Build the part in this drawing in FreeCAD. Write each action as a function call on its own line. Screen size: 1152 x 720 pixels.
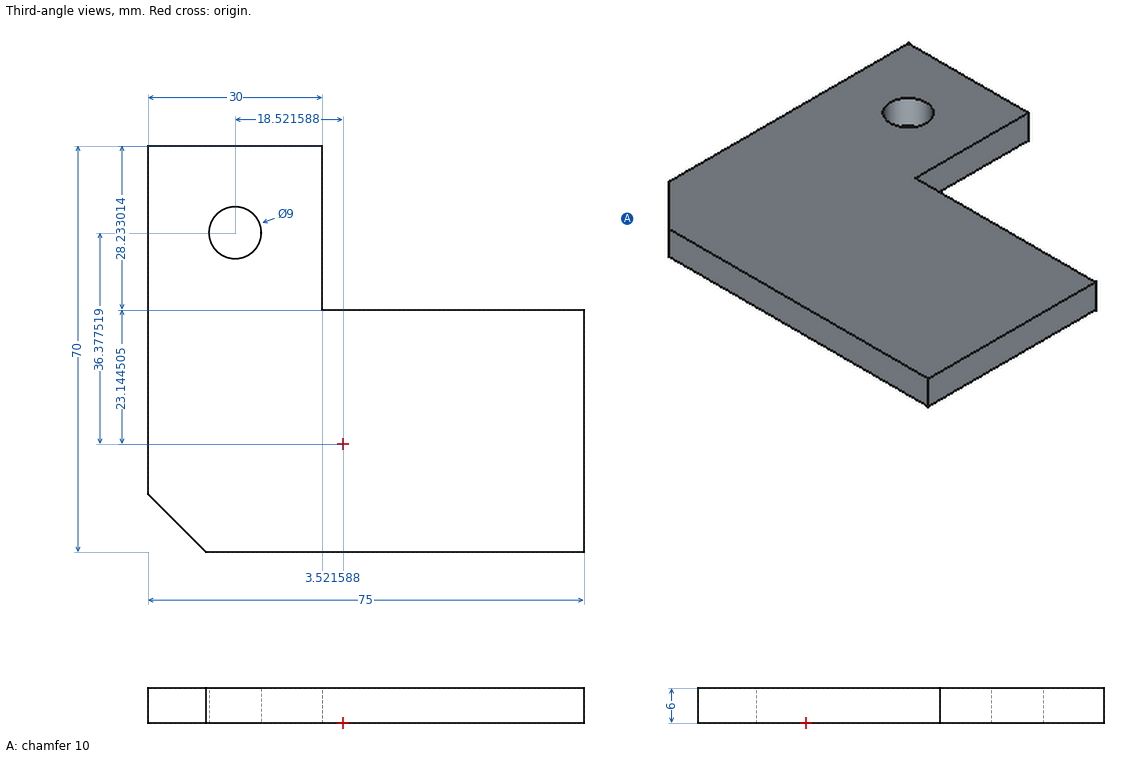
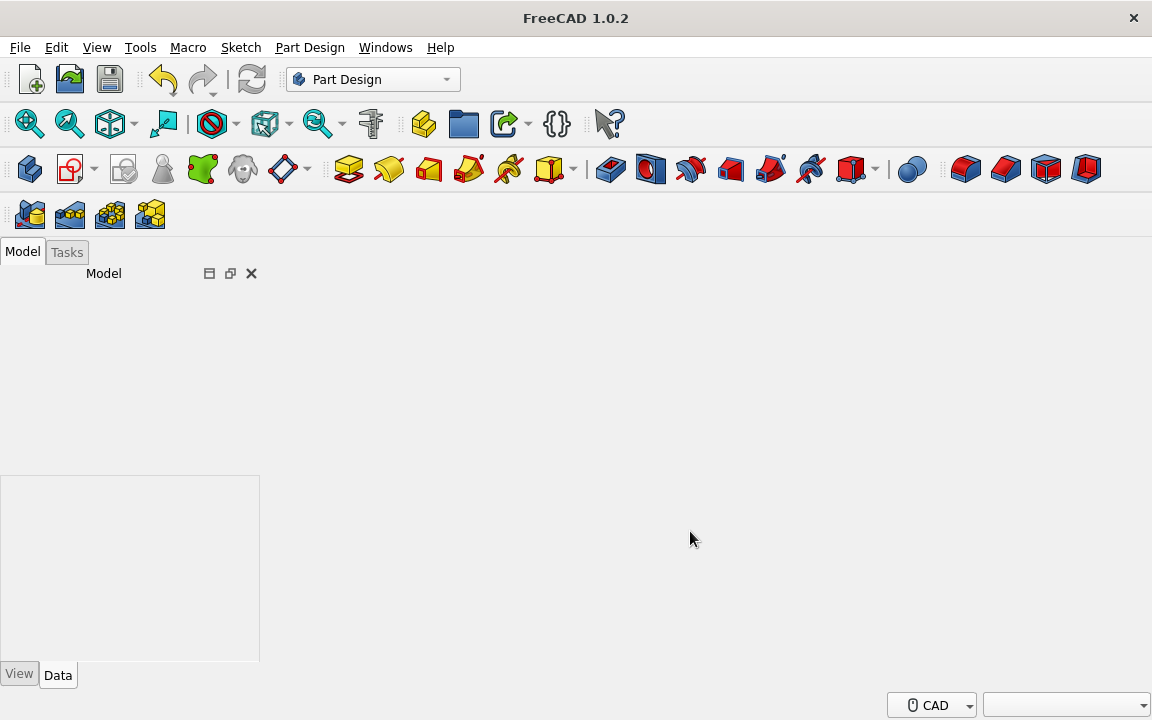
click(30, 80)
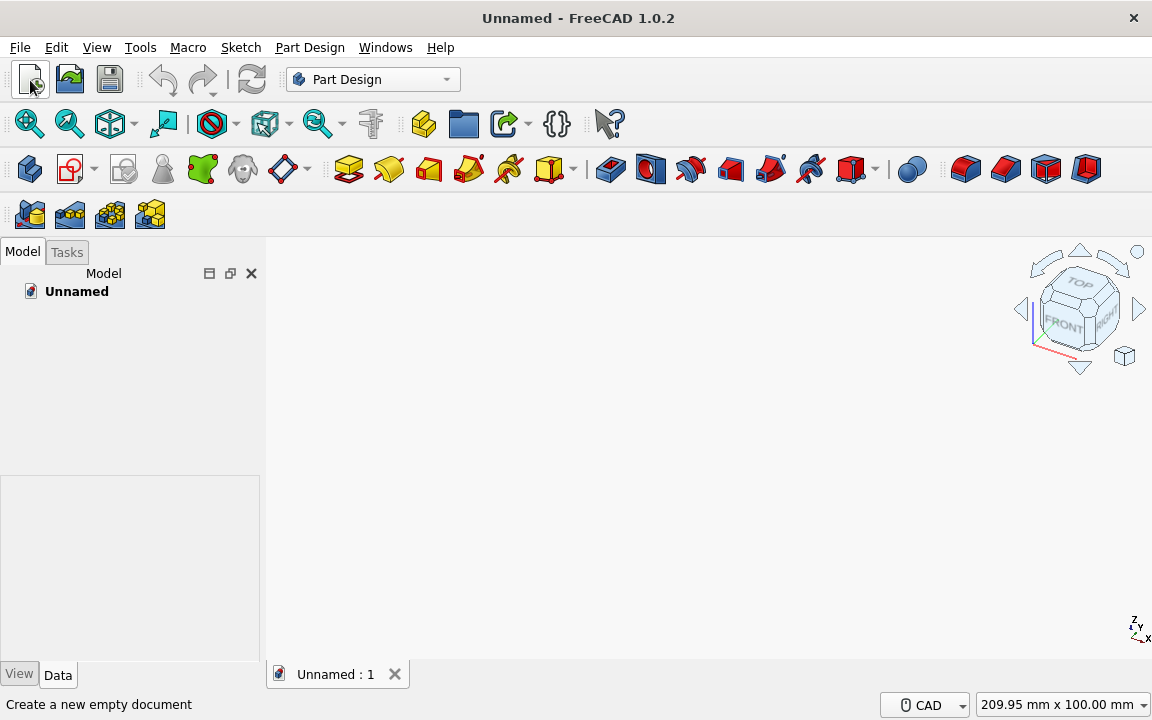
click(70, 170)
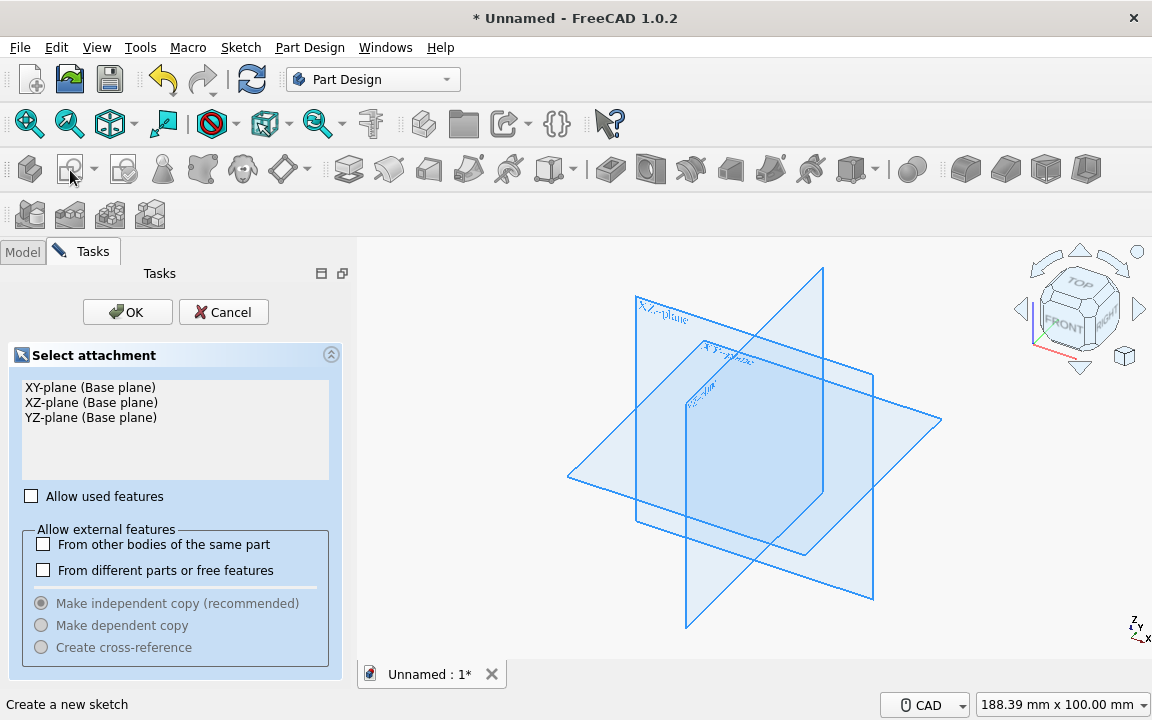
click(82, 388)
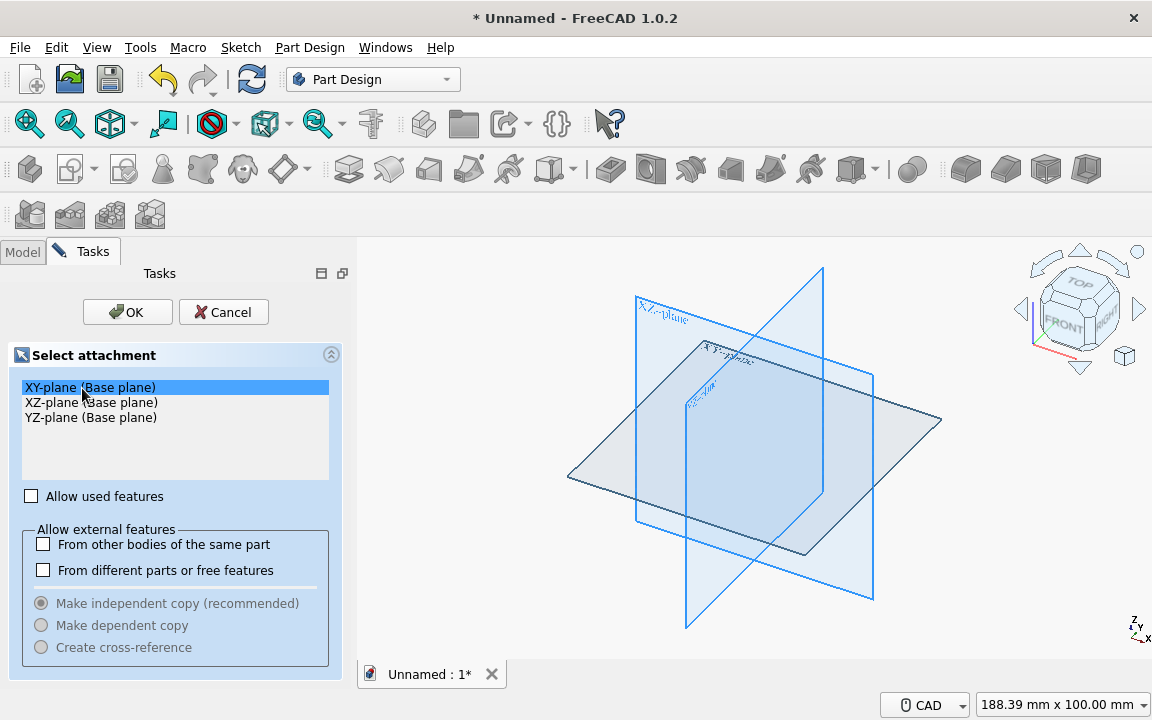
click(128, 312)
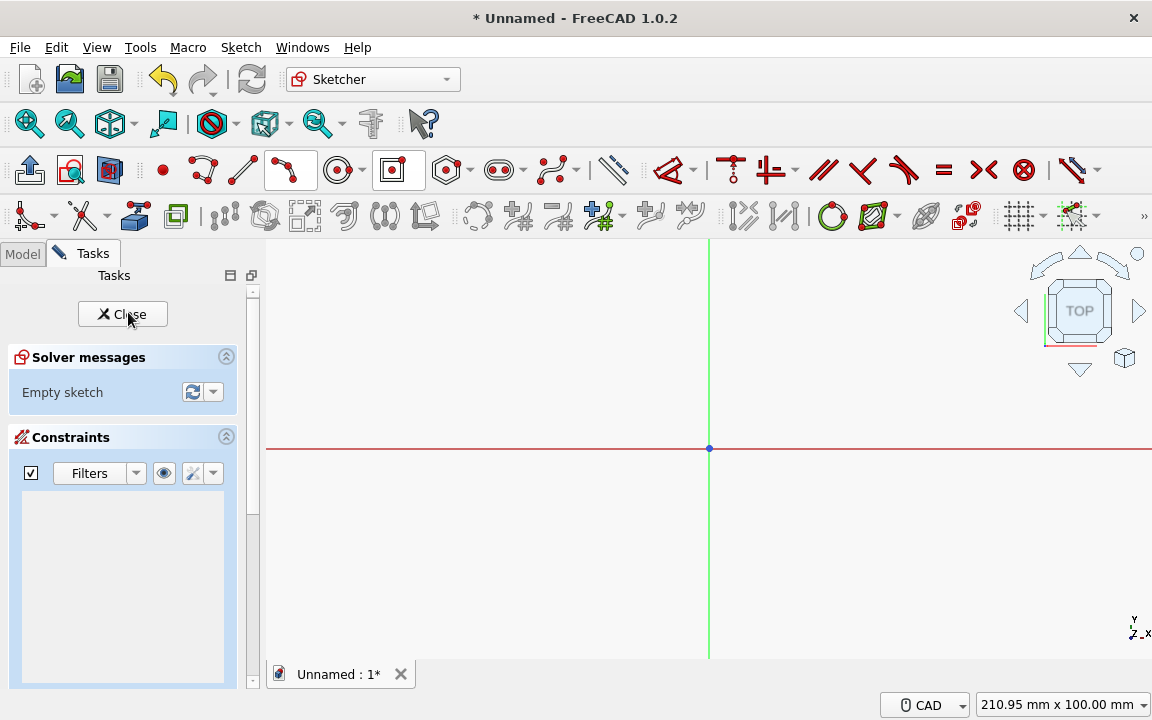
scroll(294, 631, down, 1)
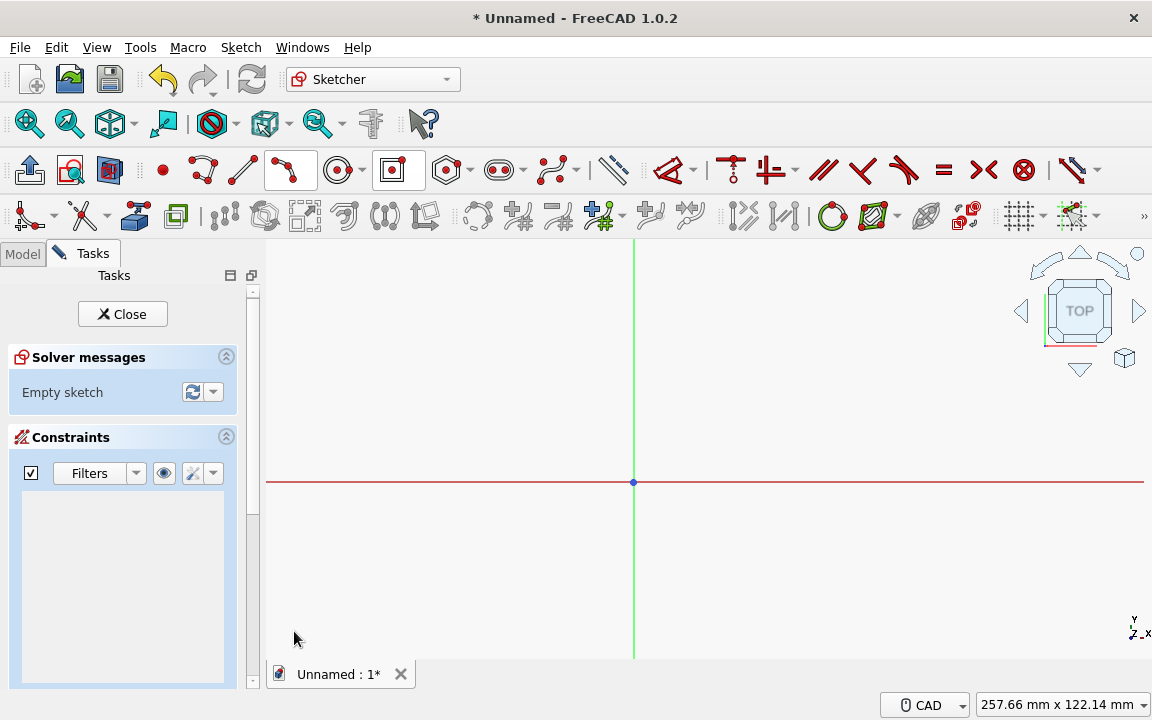
click(204, 170)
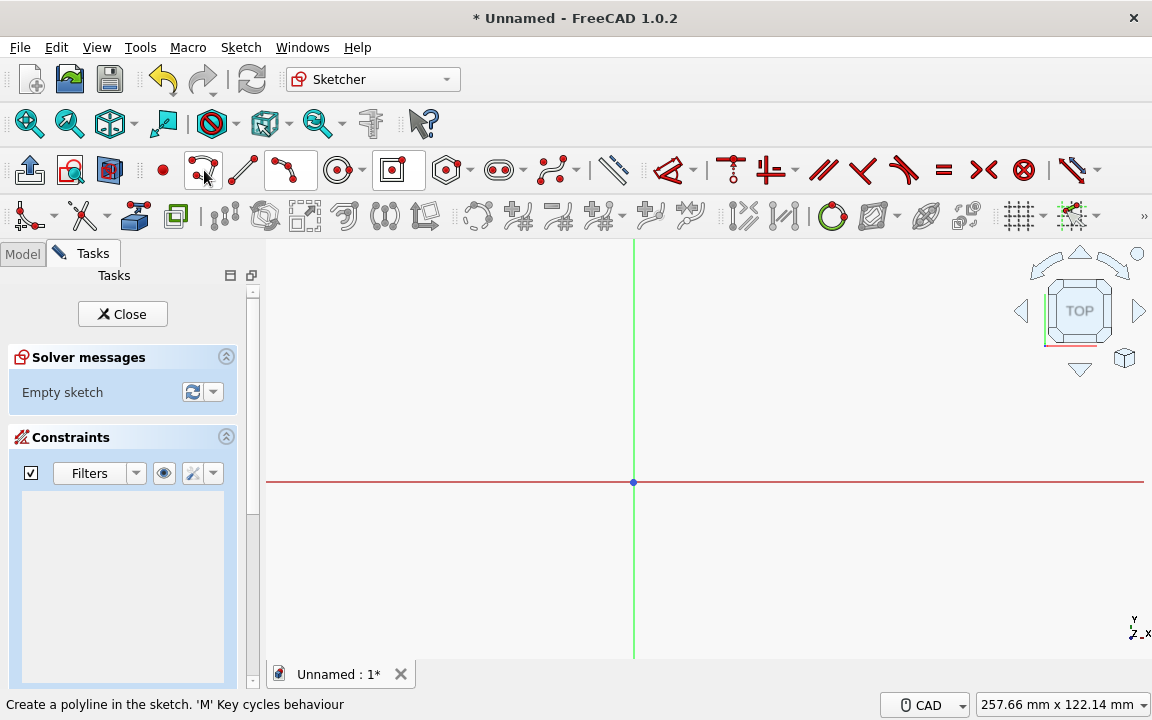
scroll(622, 403, up, 2)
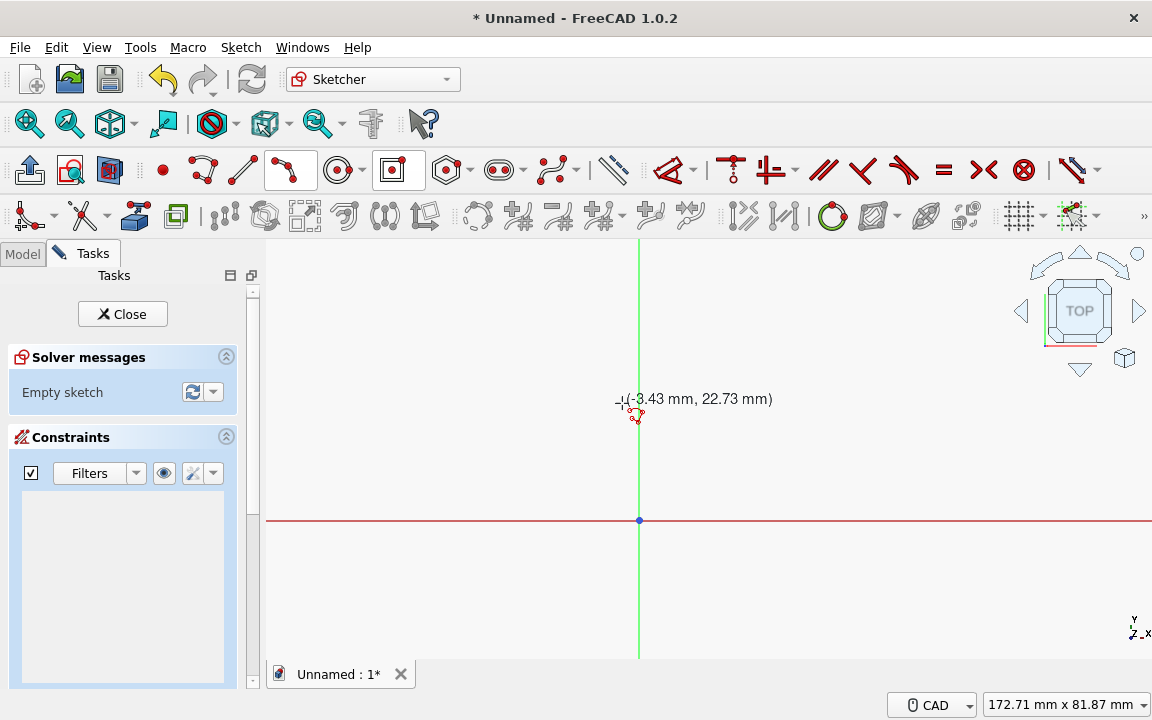
click(621, 402)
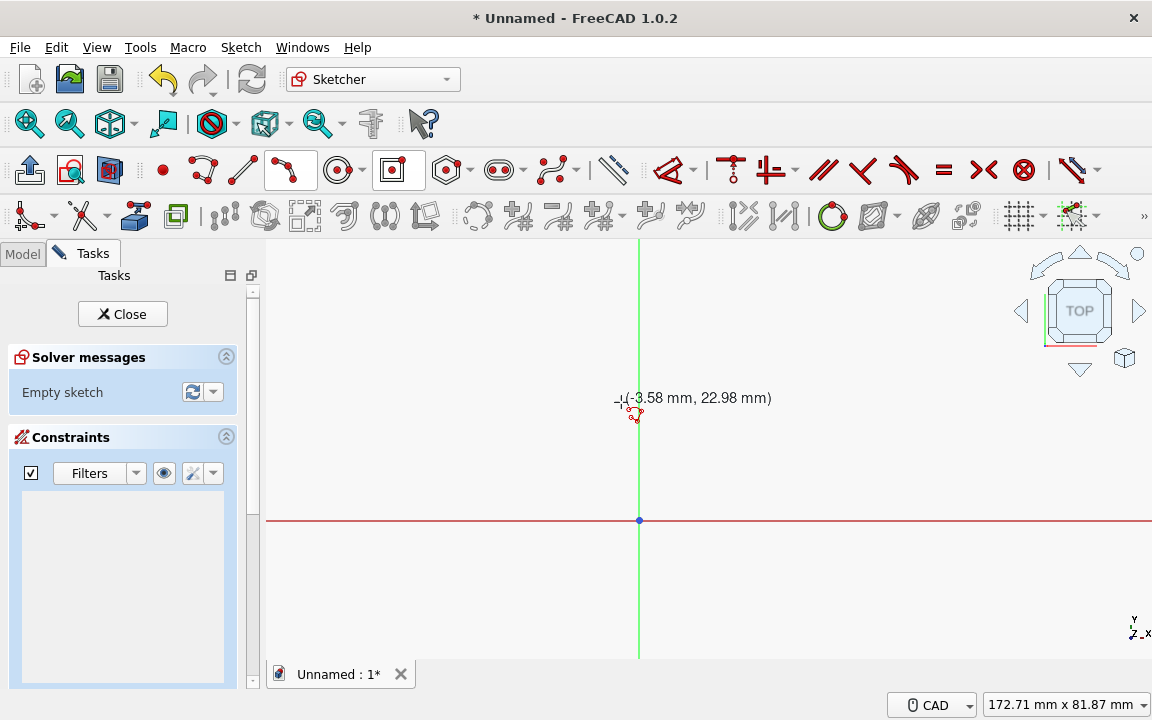
scroll(601, 474, down, 2)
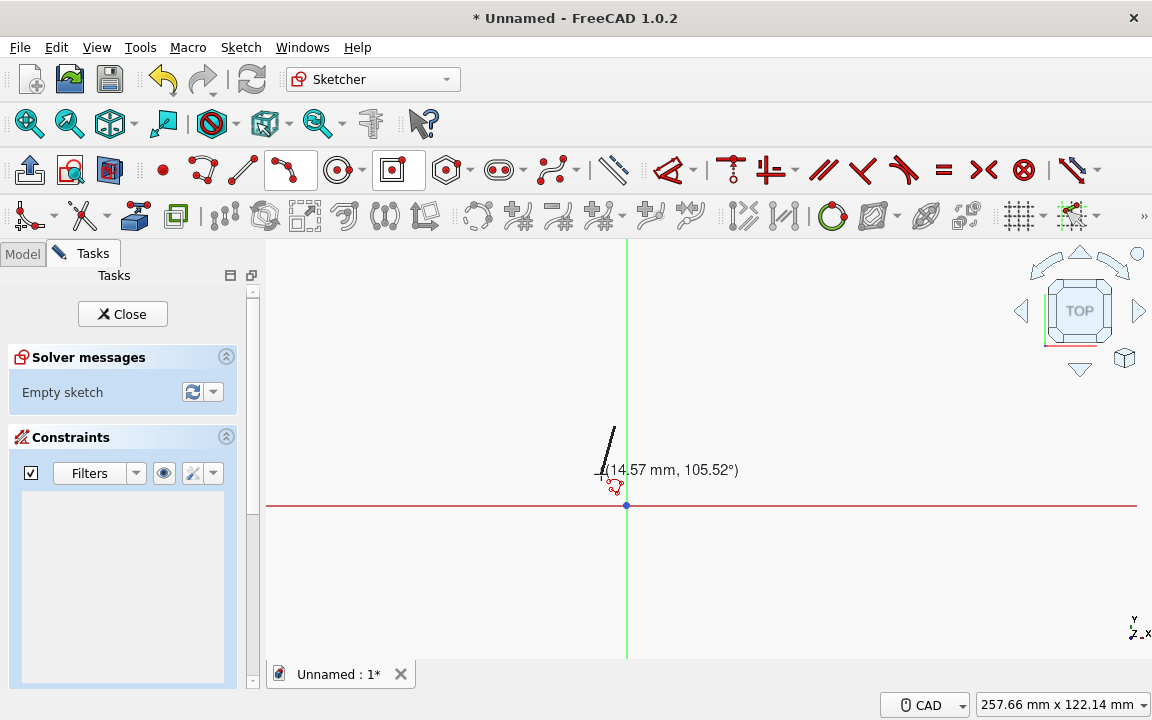
scroll(615, 329, up, 2)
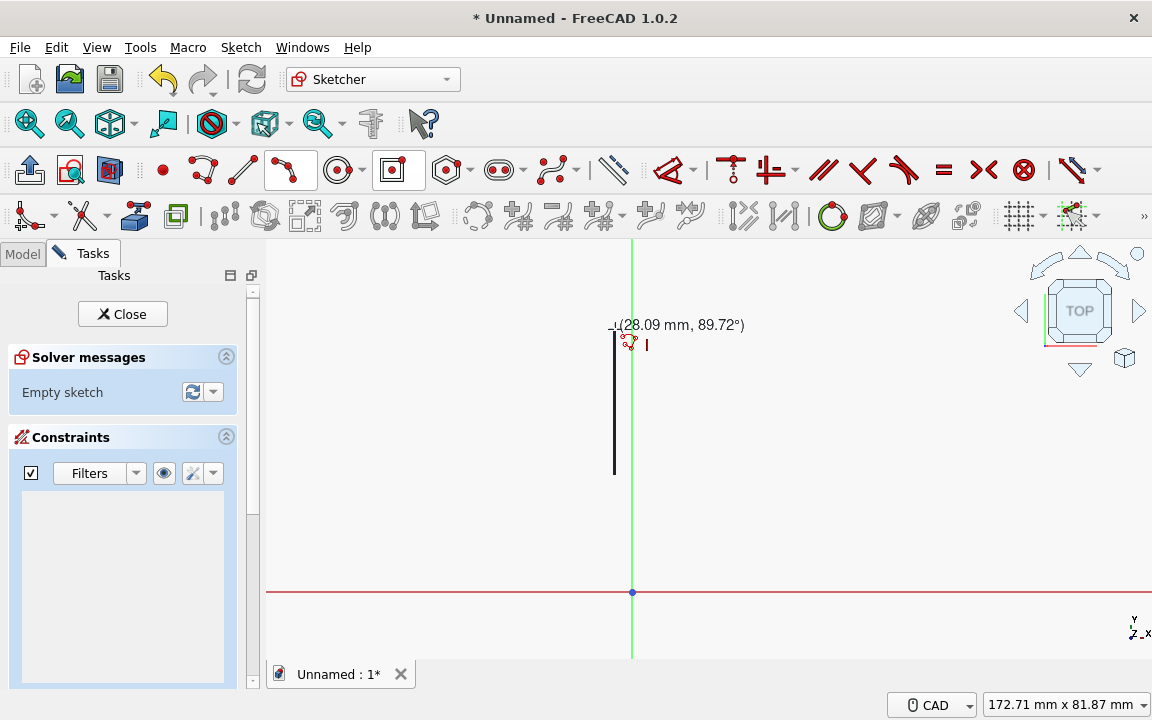
click(614, 329)
click(461, 329)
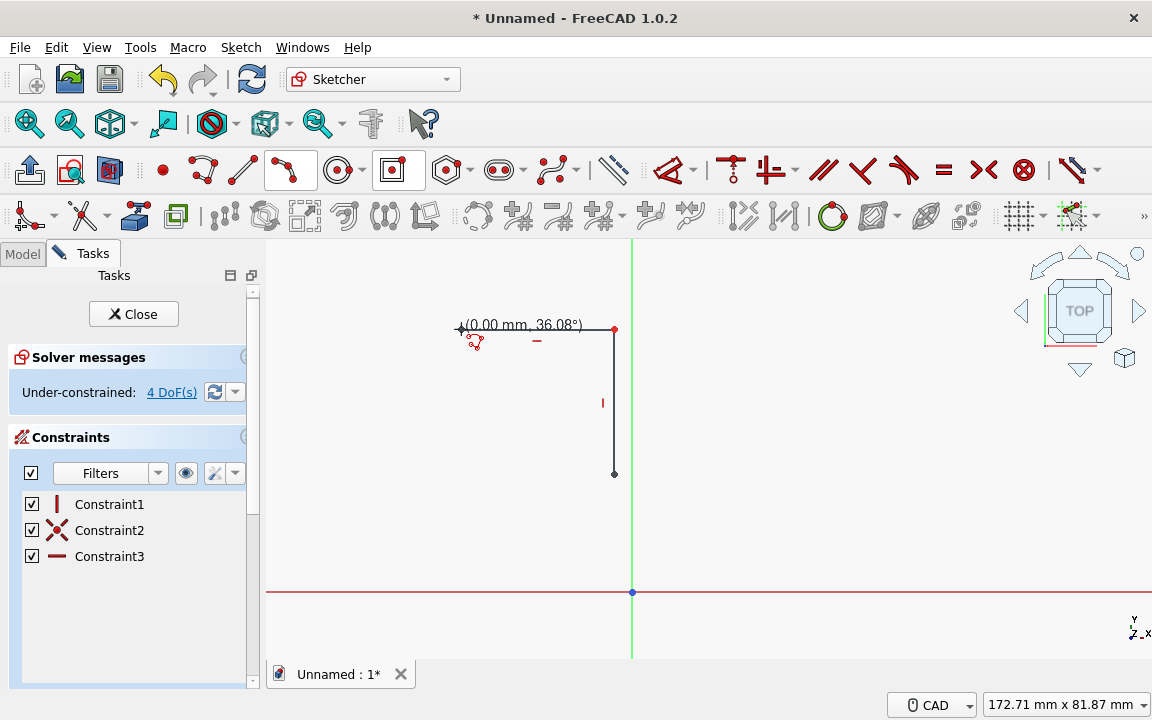
scroll(615, 328, down, 2)